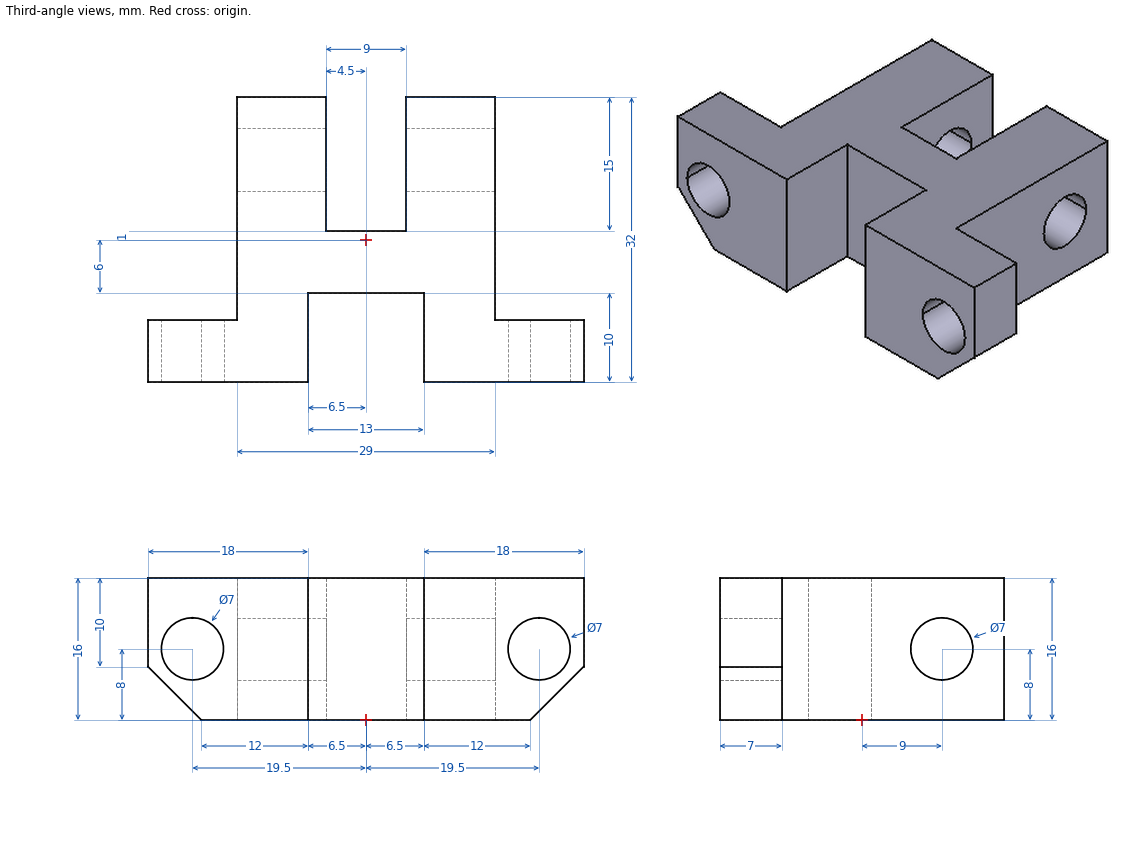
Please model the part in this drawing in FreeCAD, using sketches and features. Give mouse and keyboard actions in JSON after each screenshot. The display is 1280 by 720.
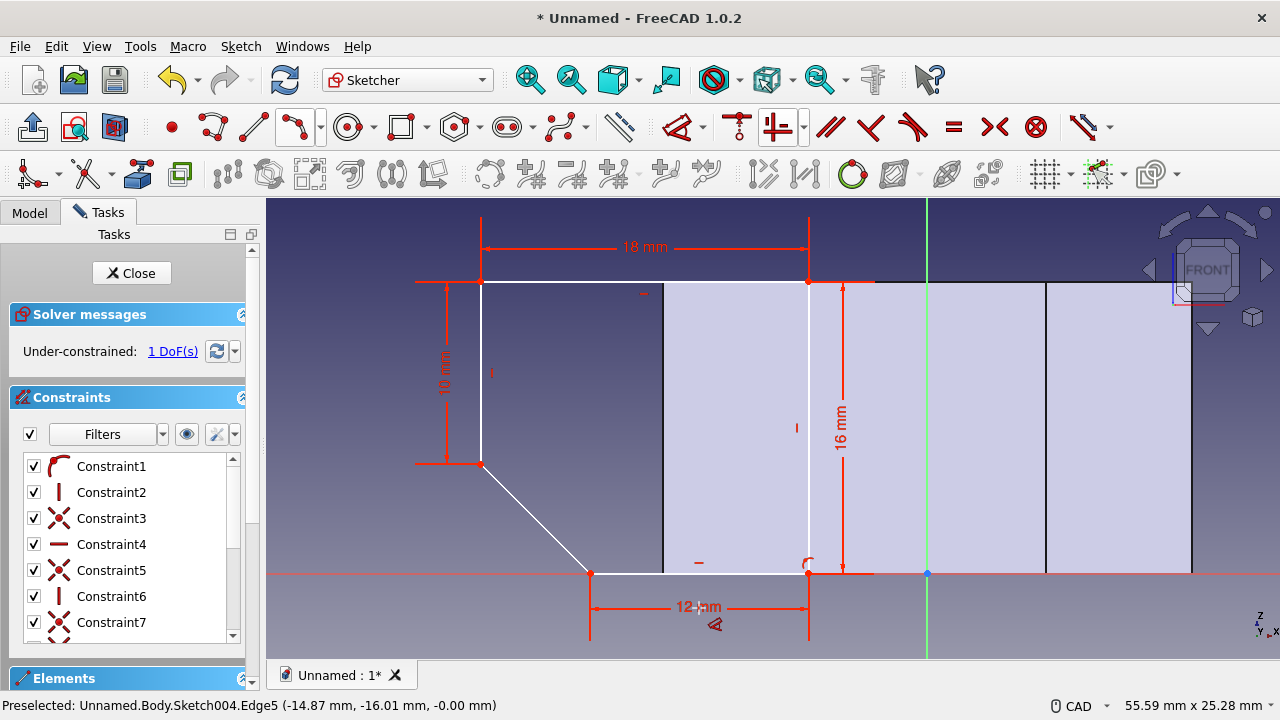
{"action": "left_click", "coordinate": [809, 574]}
{"action": "left_click", "coordinate": [868, 608]}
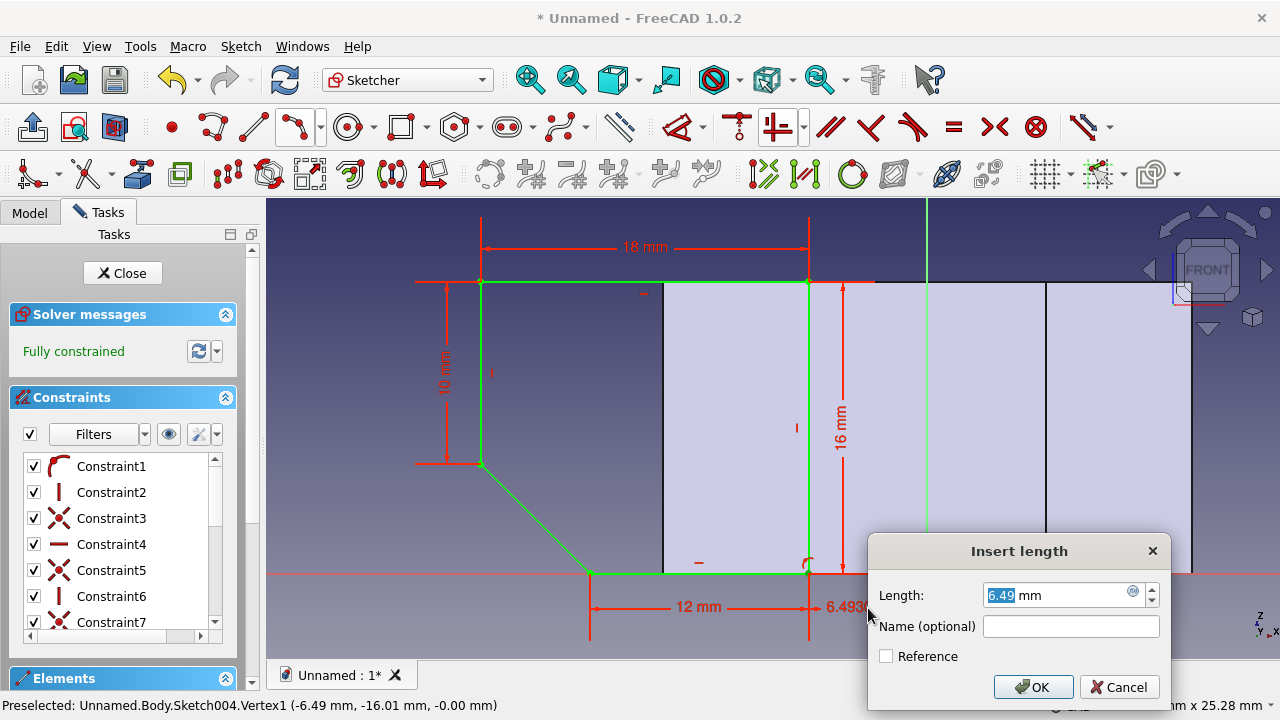
{"action": "type", "text": "6.5"}
{"action": "key", "text": "Return"}
{"action": "key", "text": "Escape"}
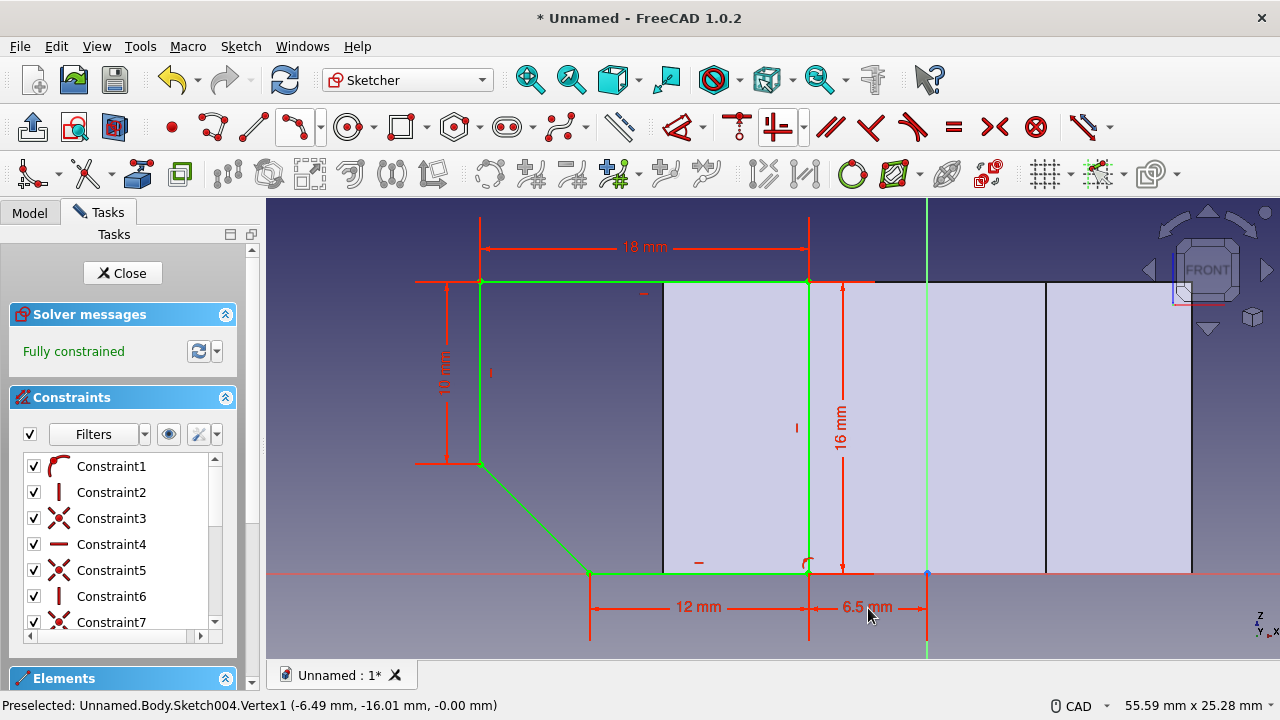
{"action": "left_click", "coordinate": [123, 273]}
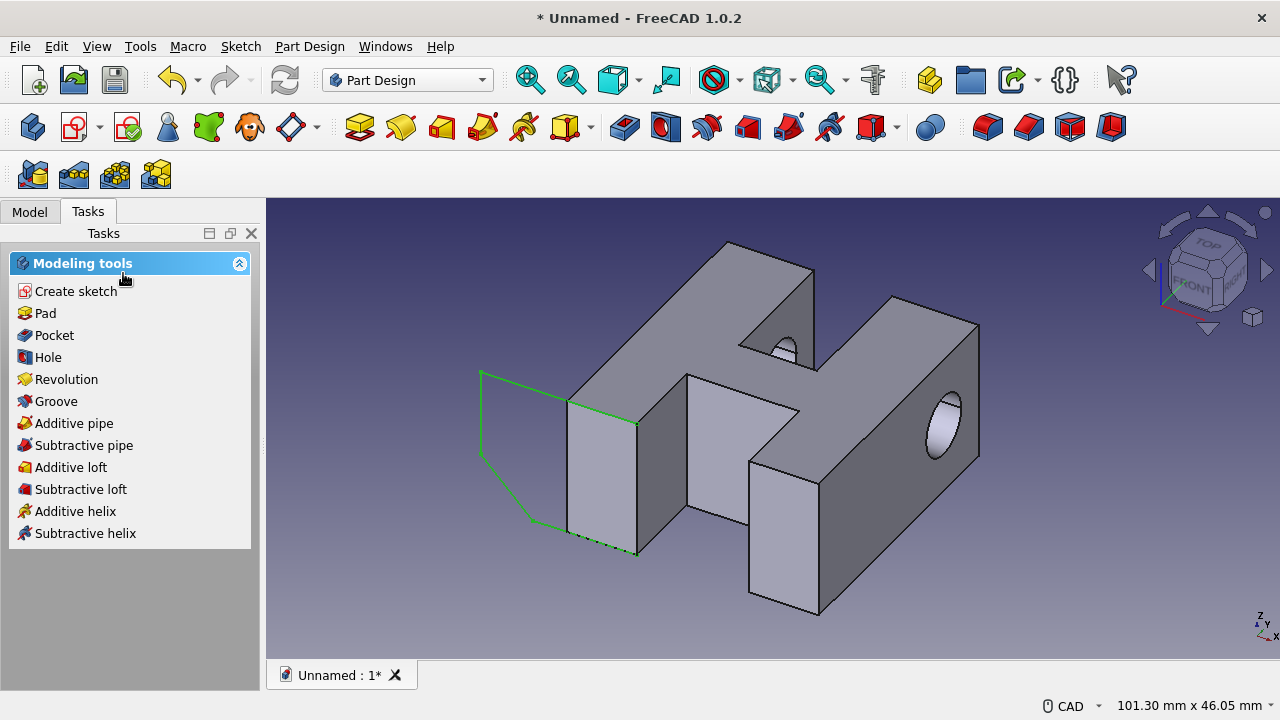
{"action": "left_click", "coordinate": [360, 128]}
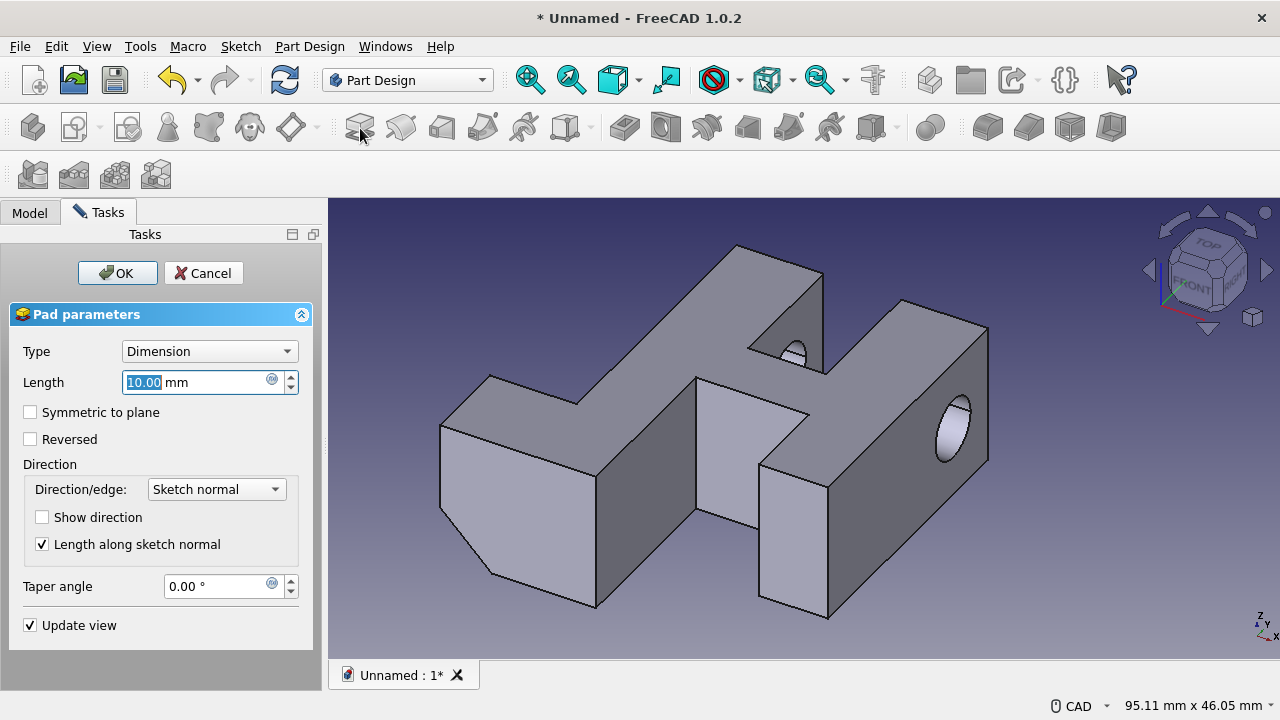
{"action": "type", "text": "7"}
{"action": "key", "text": "Tab"}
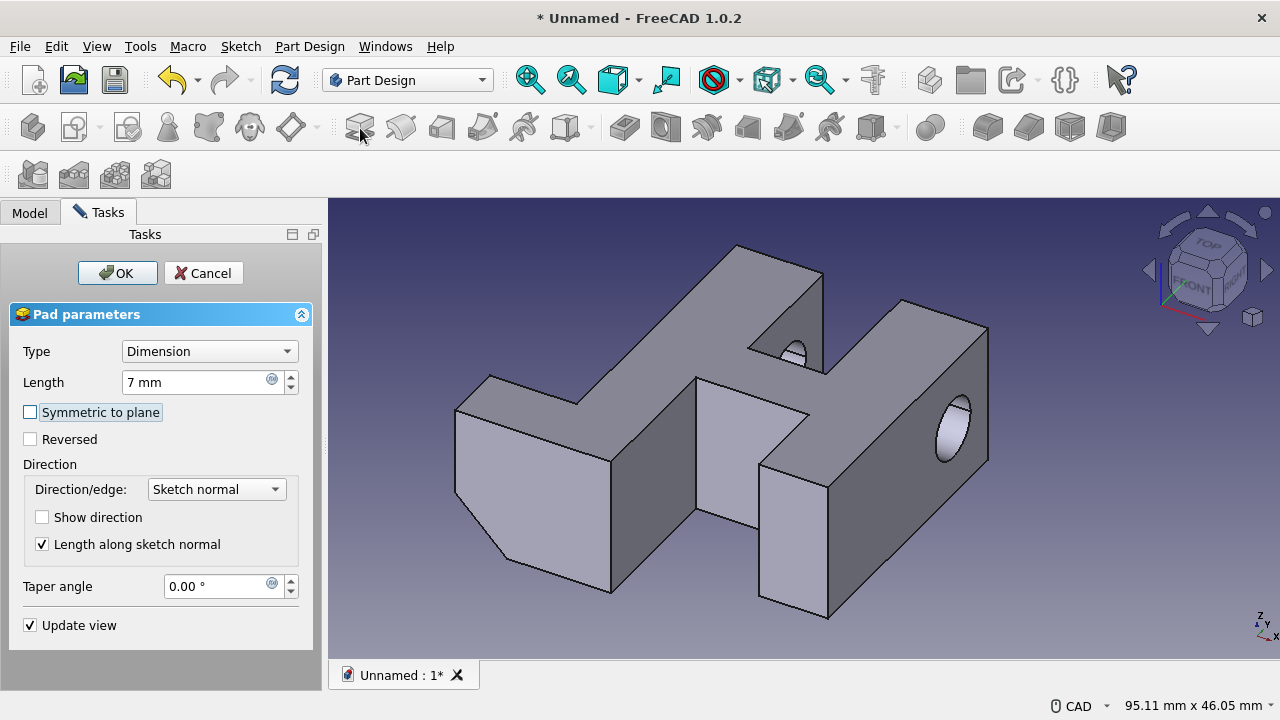
{"action": "left_click", "coordinate": [31, 439]}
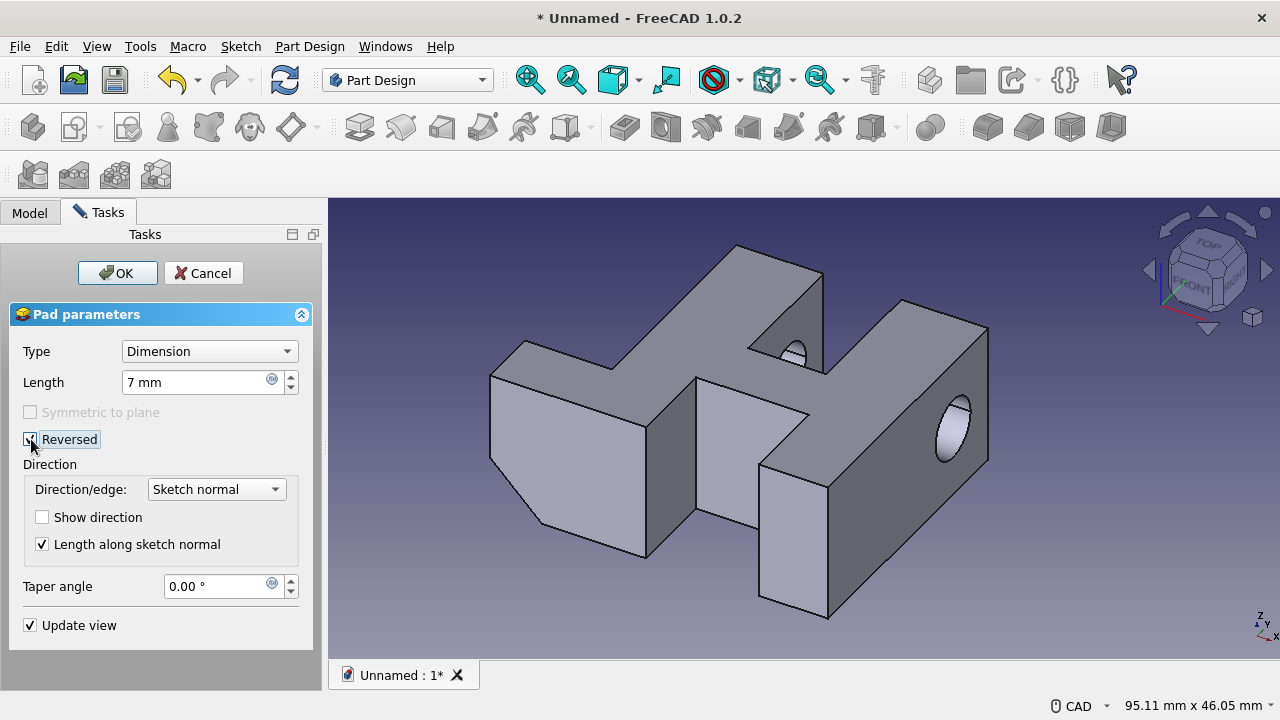
{"action": "left_click", "coordinate": [118, 273]}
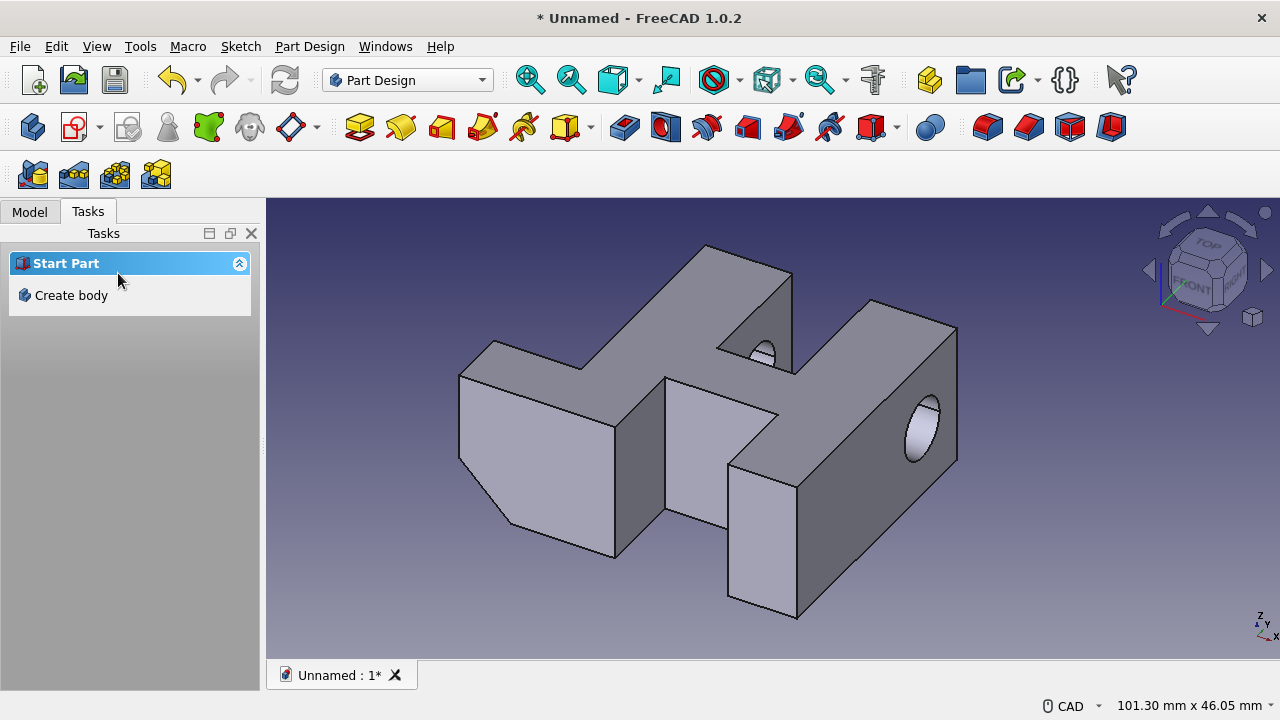
{"action": "left_click", "coordinate": [537, 466]}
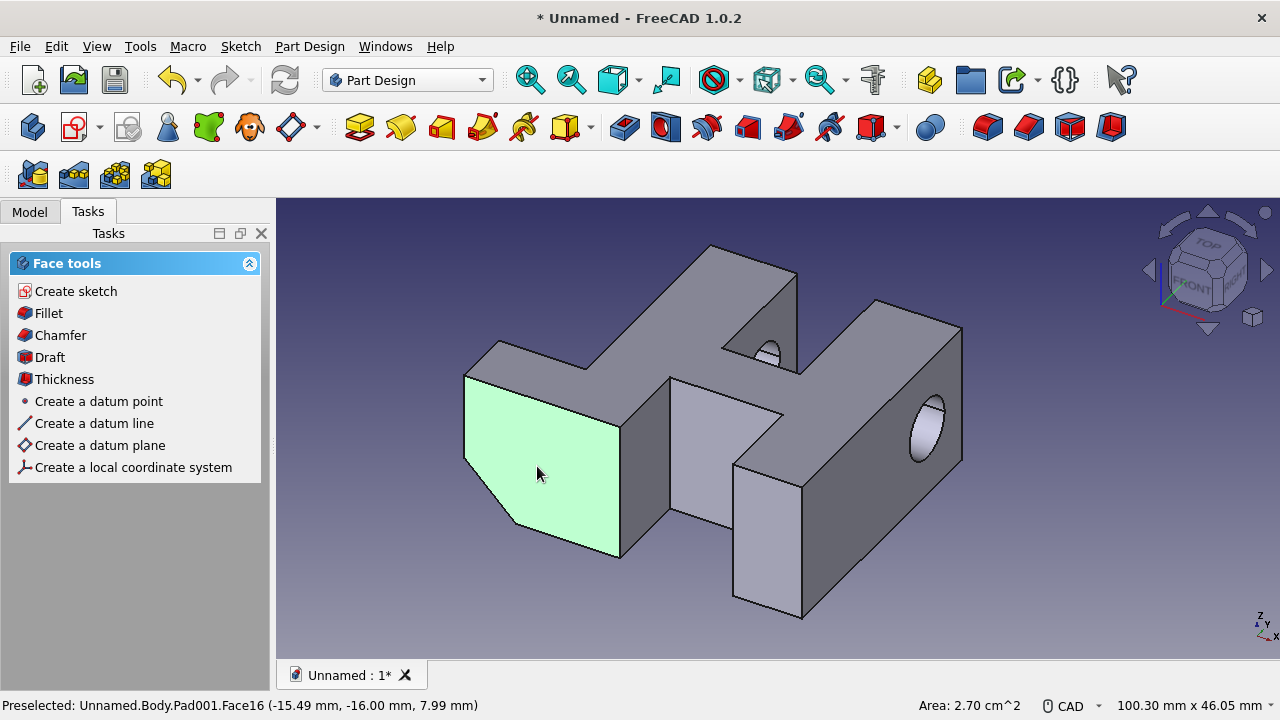
{"action": "left_click", "coordinate": [74, 128]}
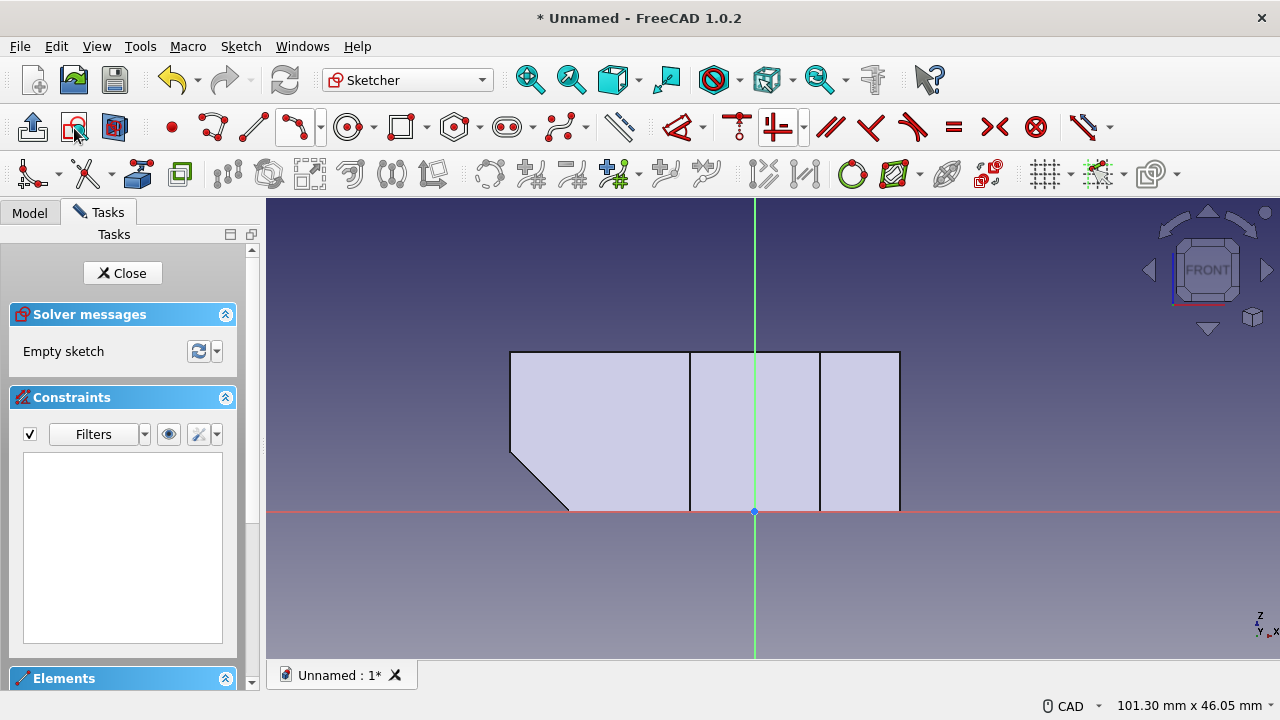
{"action": "scroll", "coordinate": [1088, 435], "scroll_direction": "up", "scroll_amount": 3}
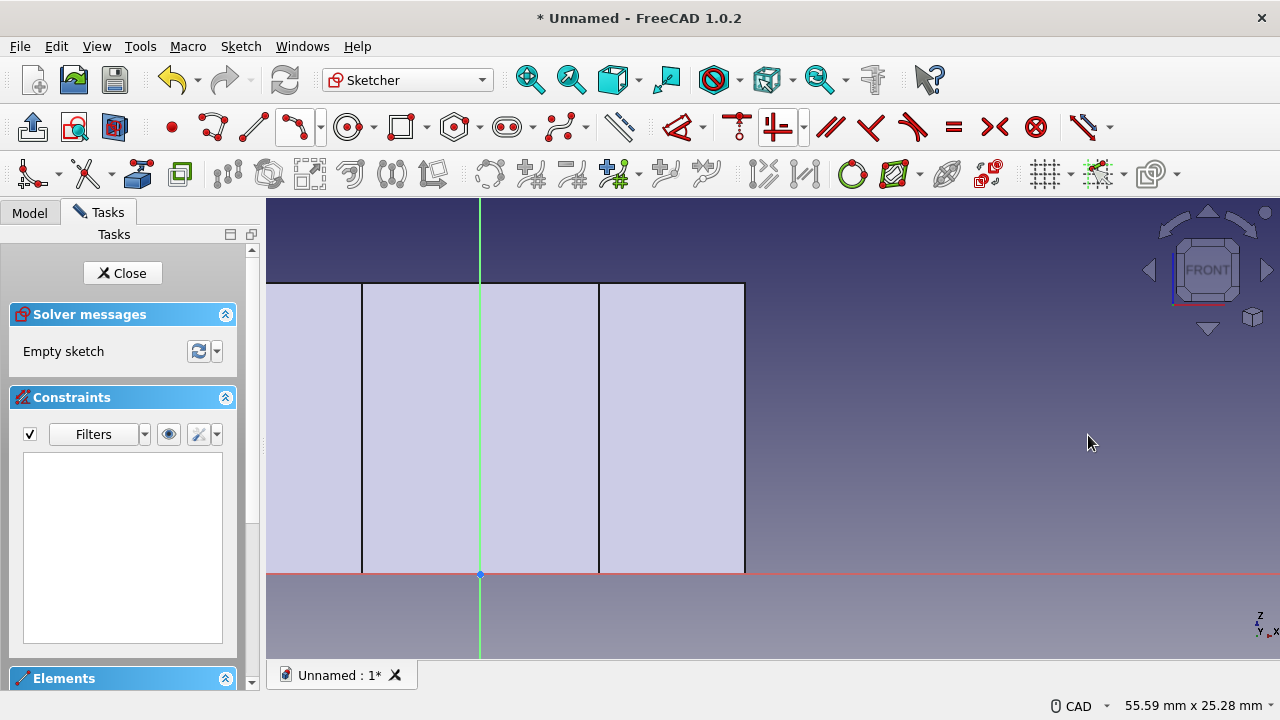
{"action": "left_click", "coordinate": [213, 128]}